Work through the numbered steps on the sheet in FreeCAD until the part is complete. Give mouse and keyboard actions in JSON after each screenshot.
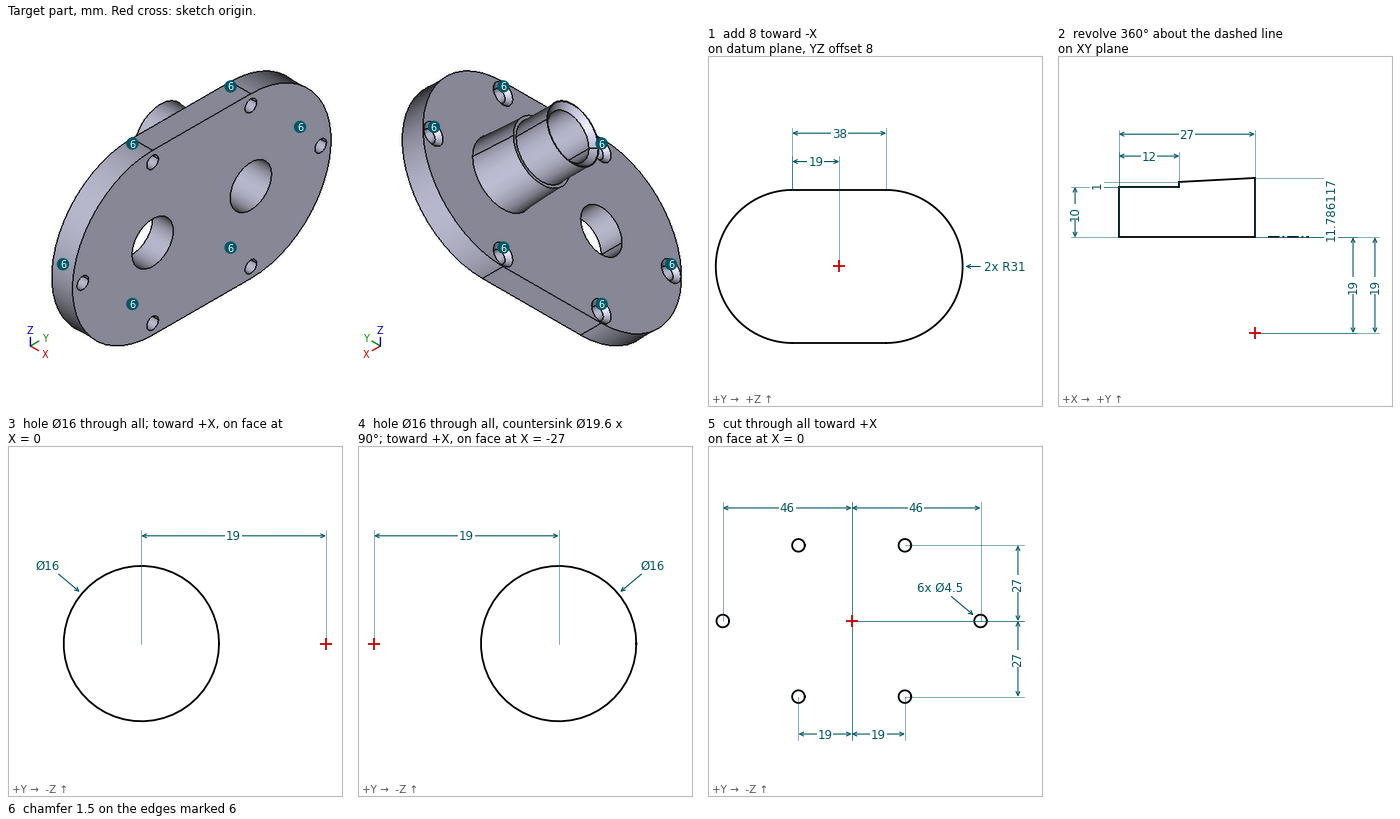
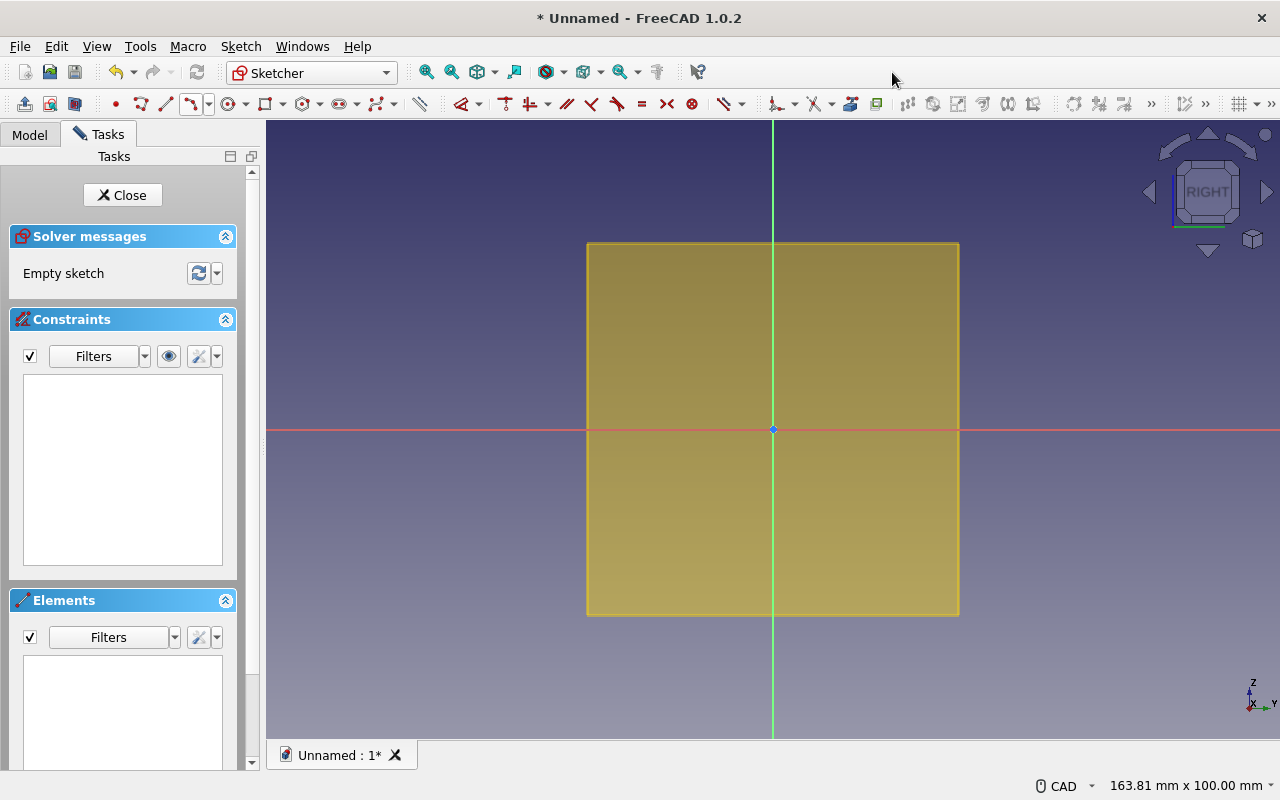
{"action": "left_click", "coordinate": [338, 104]}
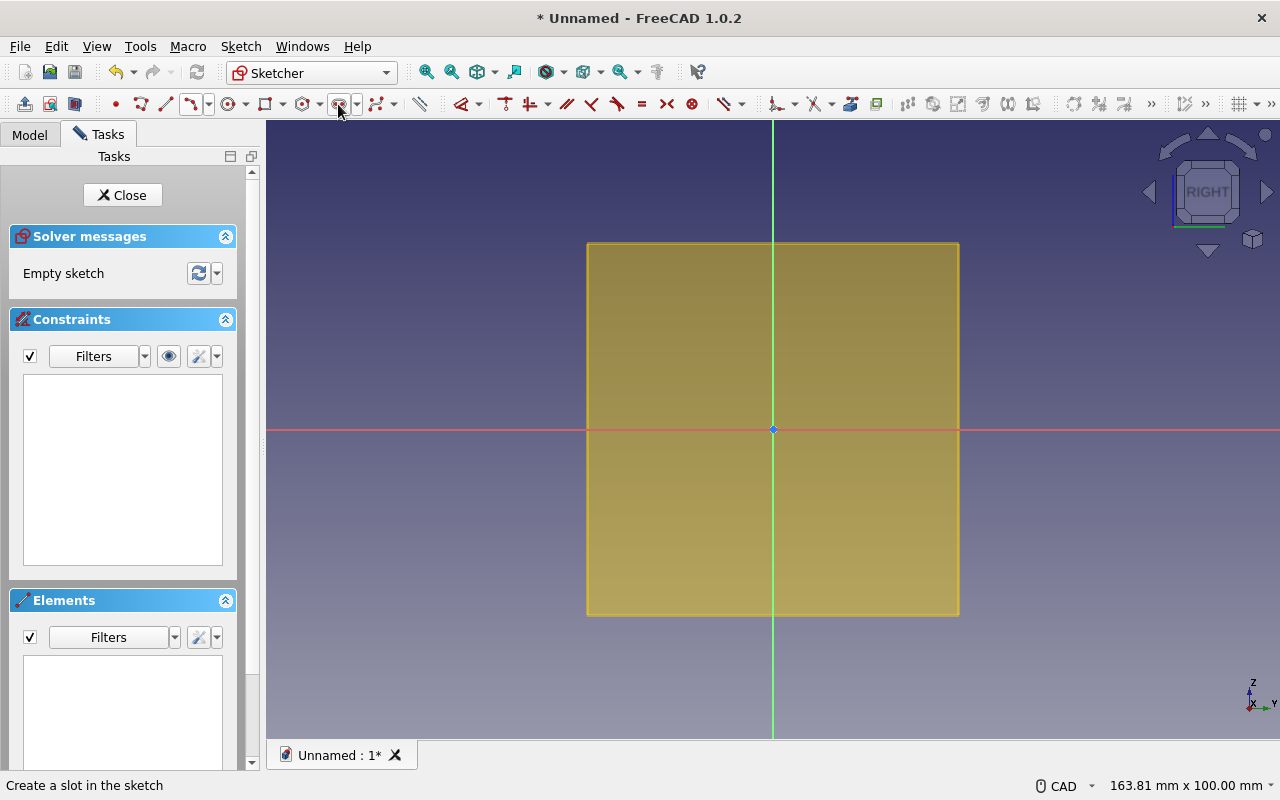
{"action": "left_click", "coordinate": [655, 430]}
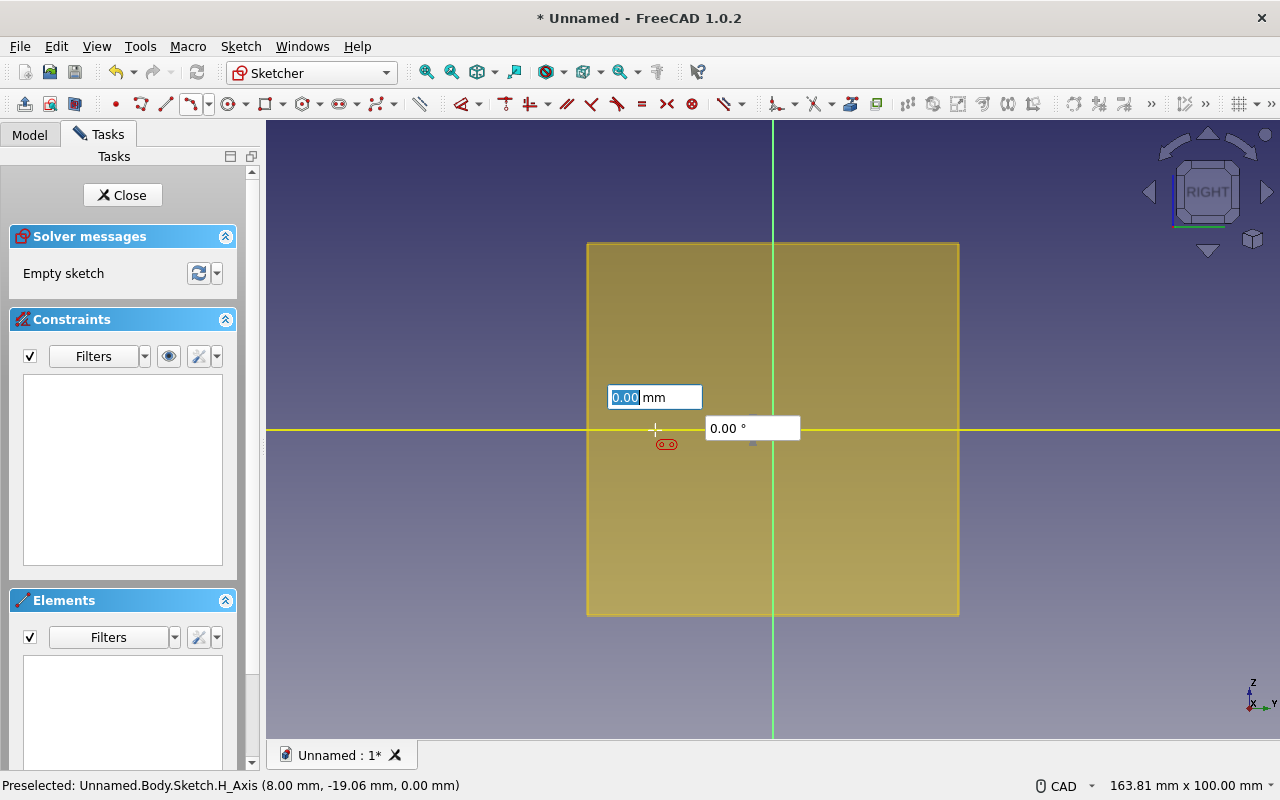
{"action": "left_click", "coordinate": [891, 420]}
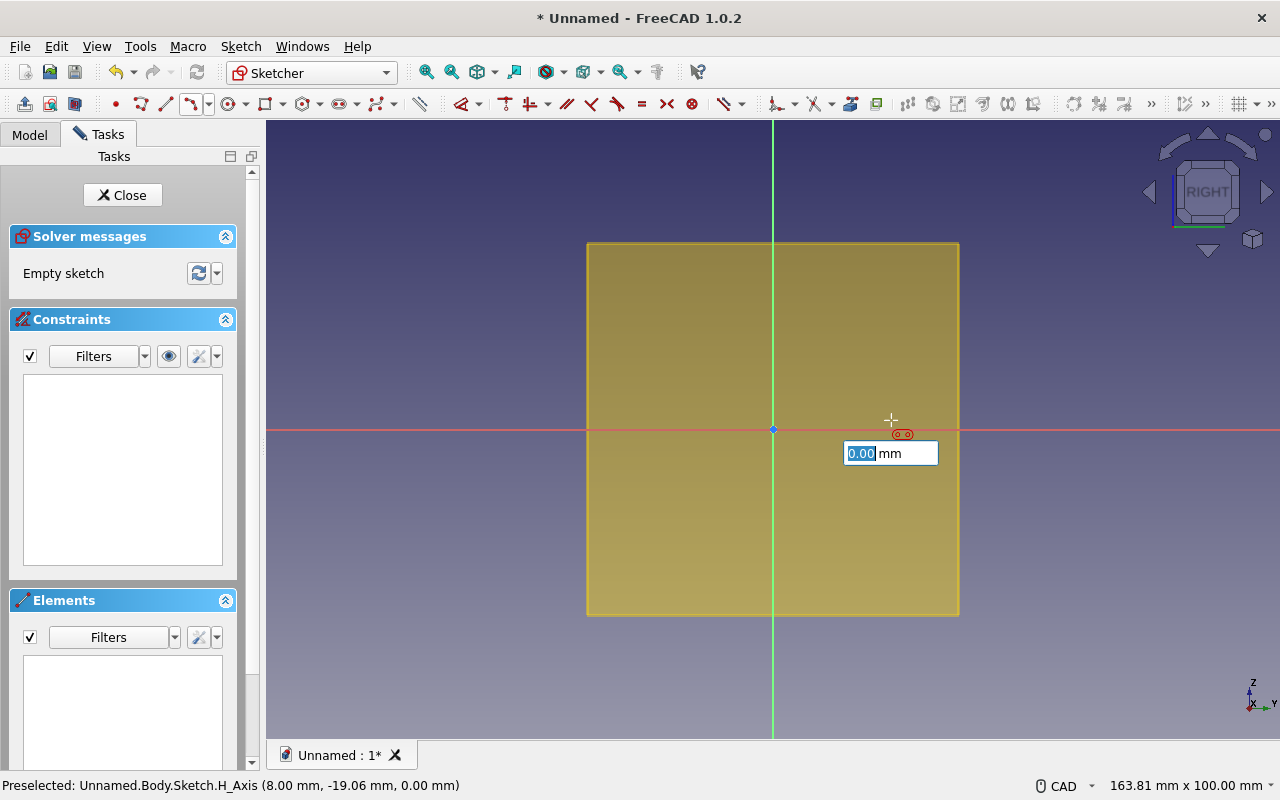
{"action": "left_click", "coordinate": [738, 621]}
{"action": "key", "text": "Escape"}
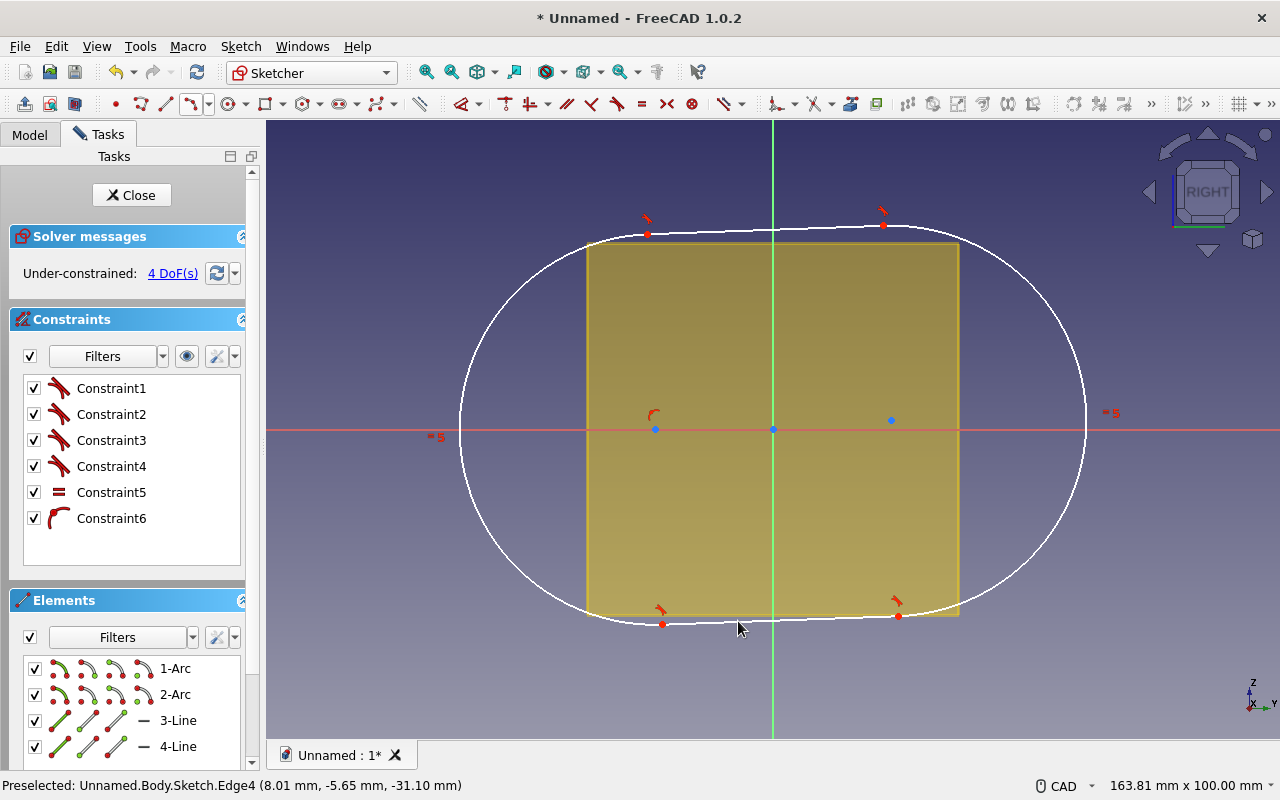
{"action": "left_click", "coordinate": [719, 232]}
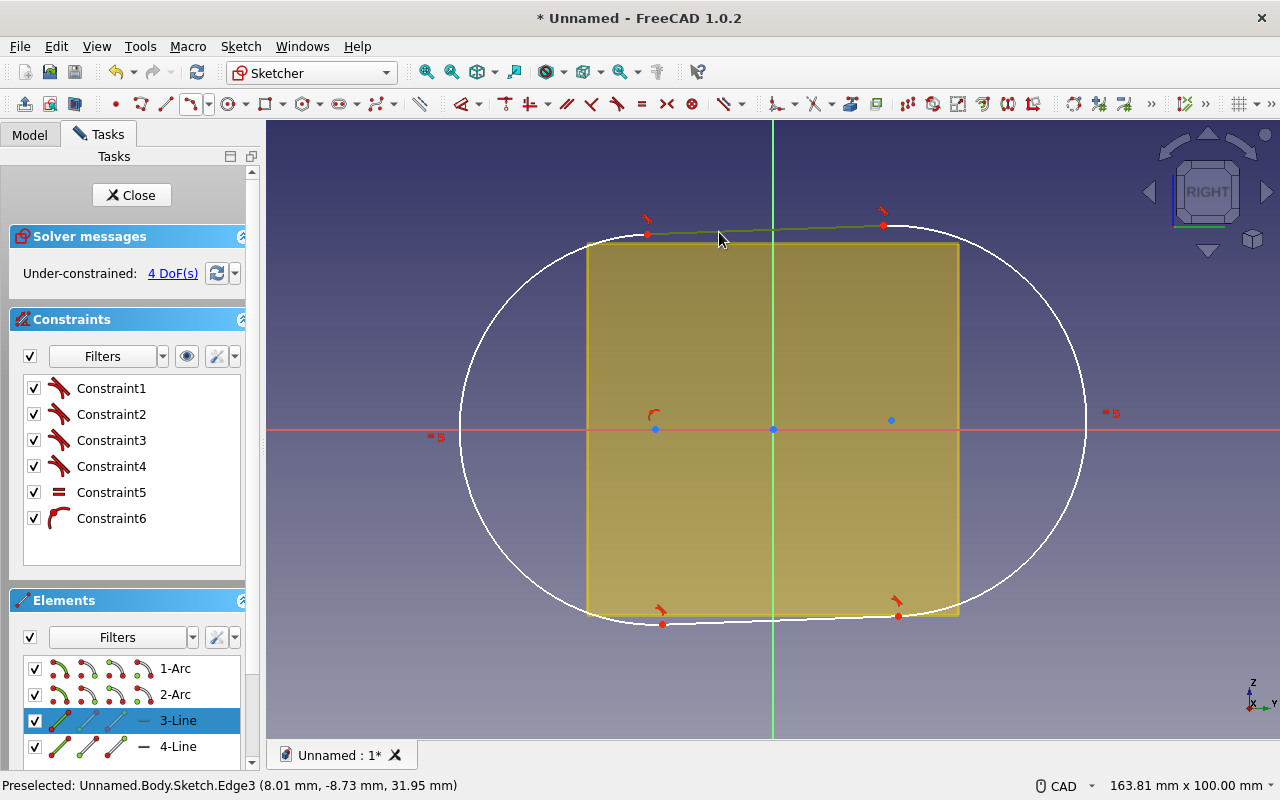
{"action": "left_click", "coordinate": [548, 104]}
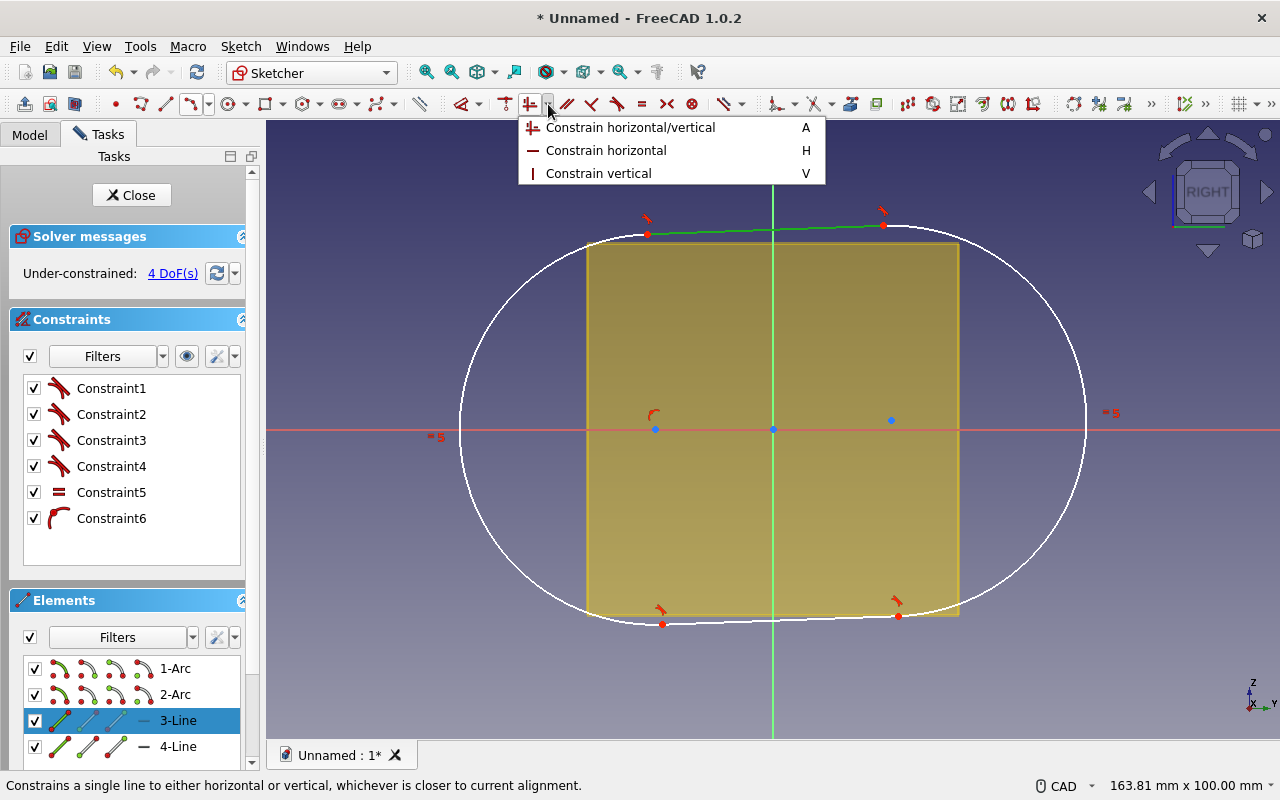
{"action": "left_click", "coordinate": [672, 150]}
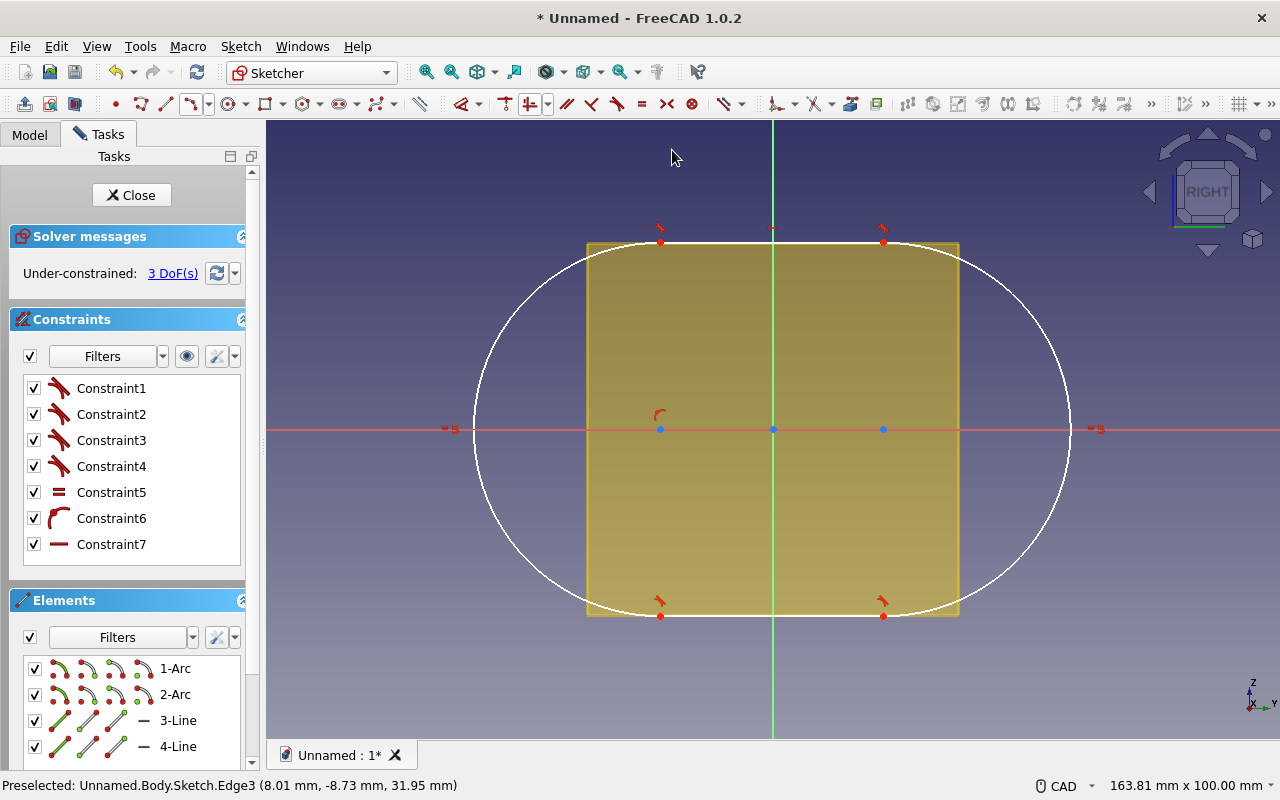
{"action": "left_click", "coordinate": [460, 104]}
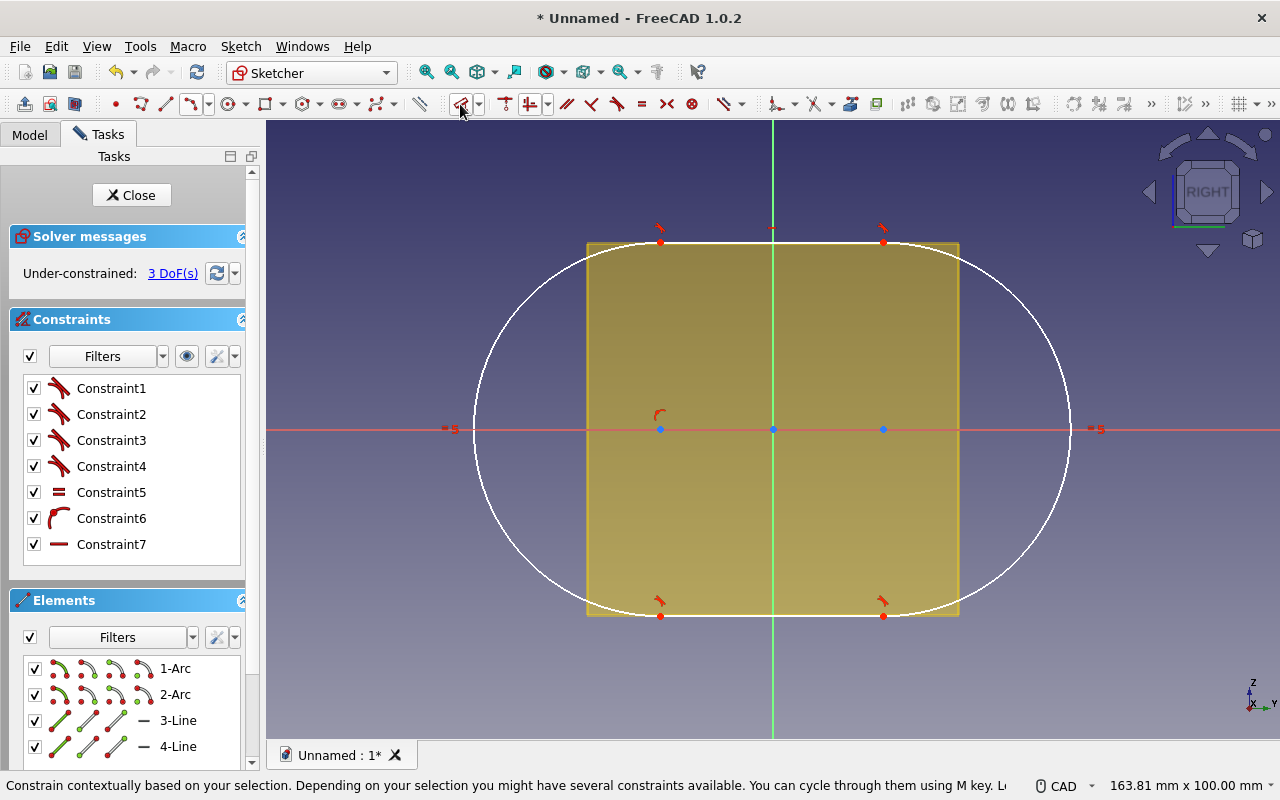
{"action": "left_click", "coordinate": [509, 320]}
{"action": "left_click", "coordinate": [483, 301]}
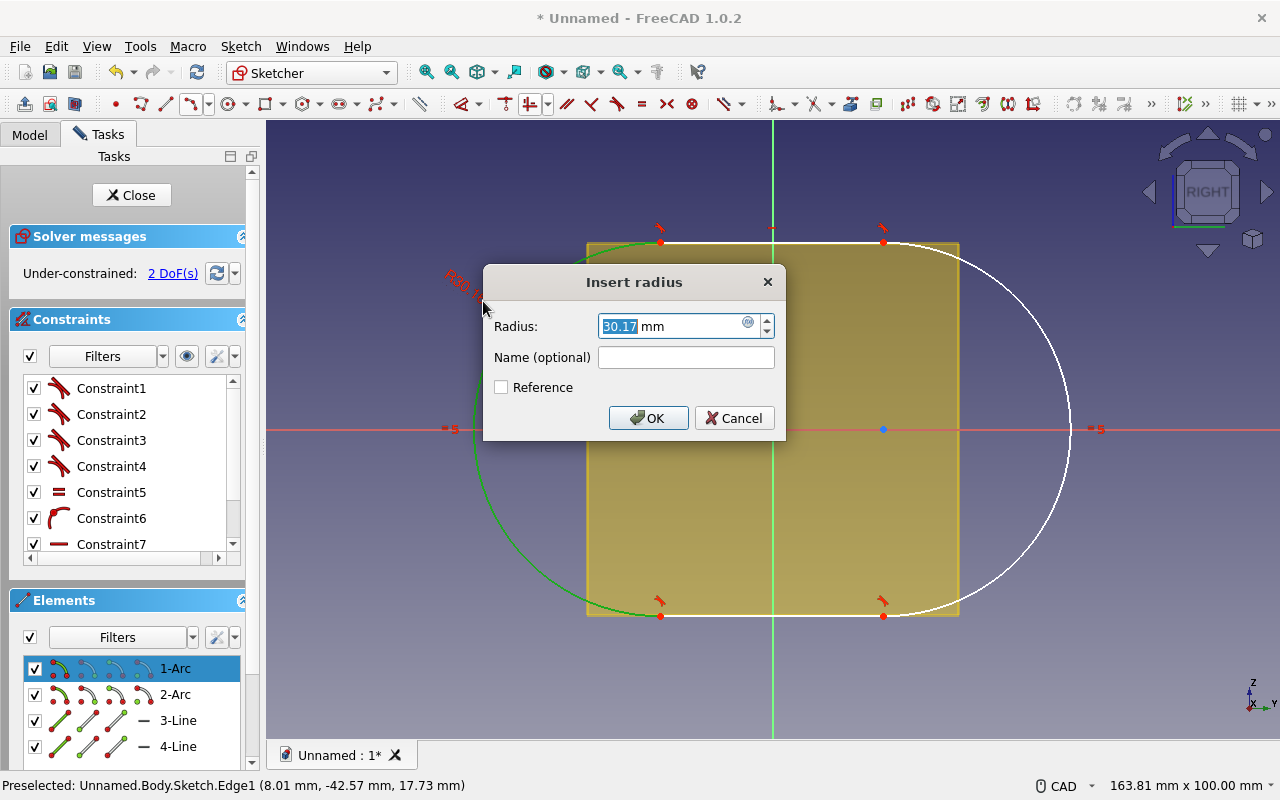
{"action": "type", "text": "31"}
{"action": "key", "text": "Return"}